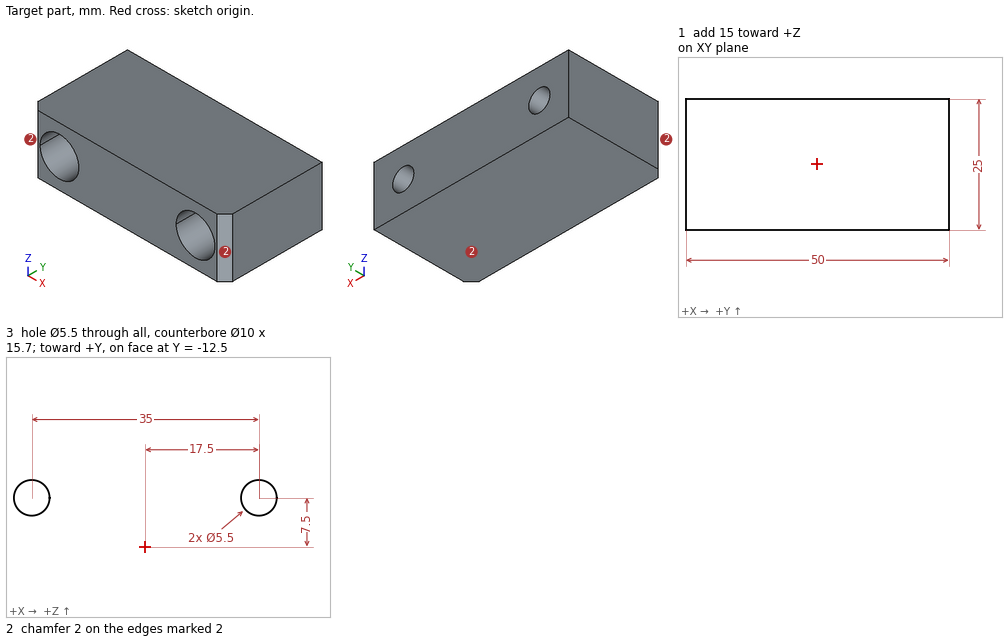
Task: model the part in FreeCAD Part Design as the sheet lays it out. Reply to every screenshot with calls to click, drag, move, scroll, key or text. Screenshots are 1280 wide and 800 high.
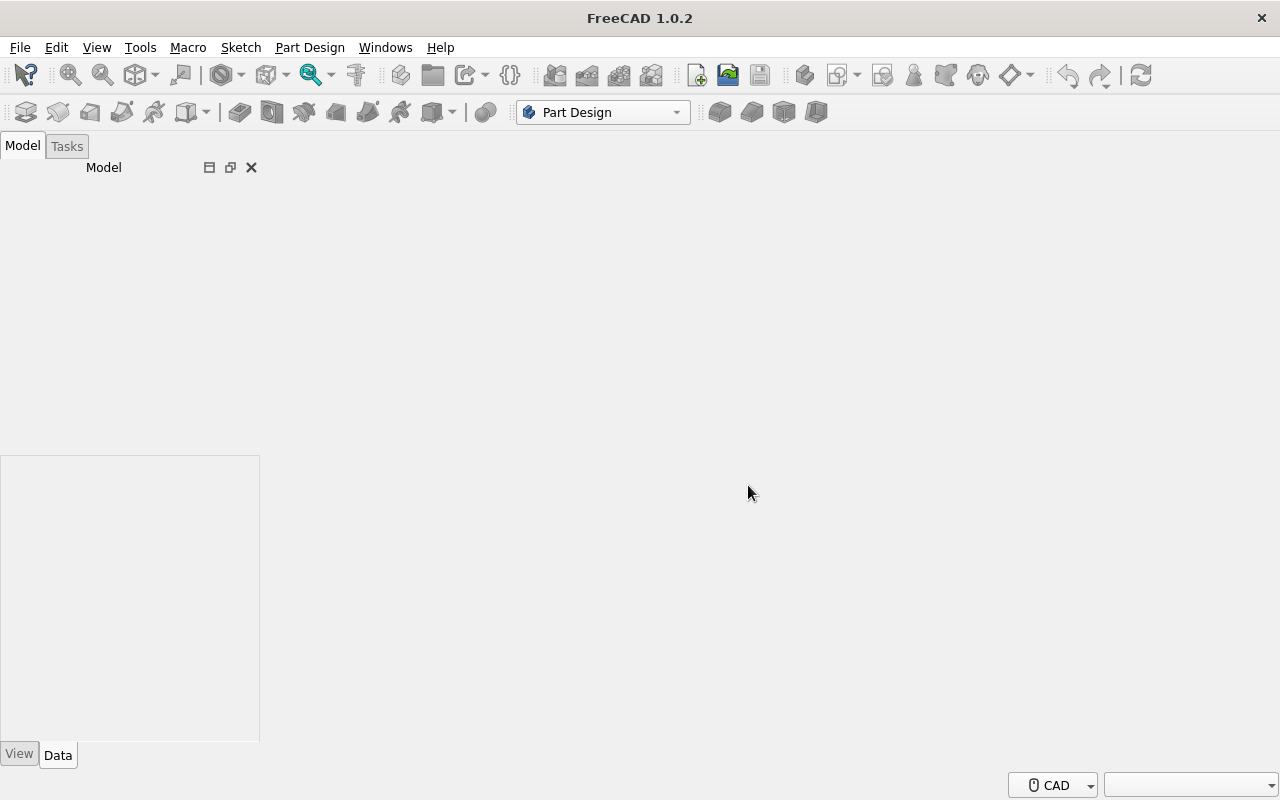
key(ctrl+n)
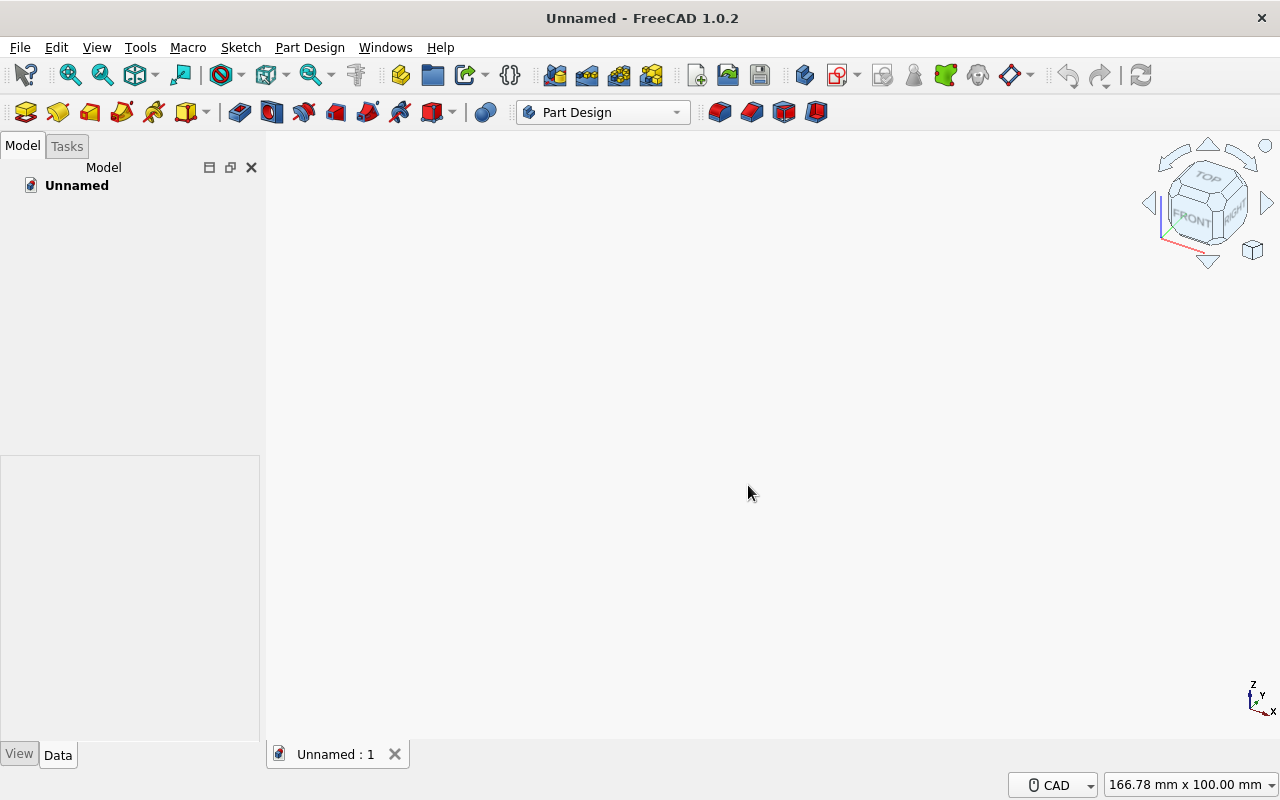
click(838, 76)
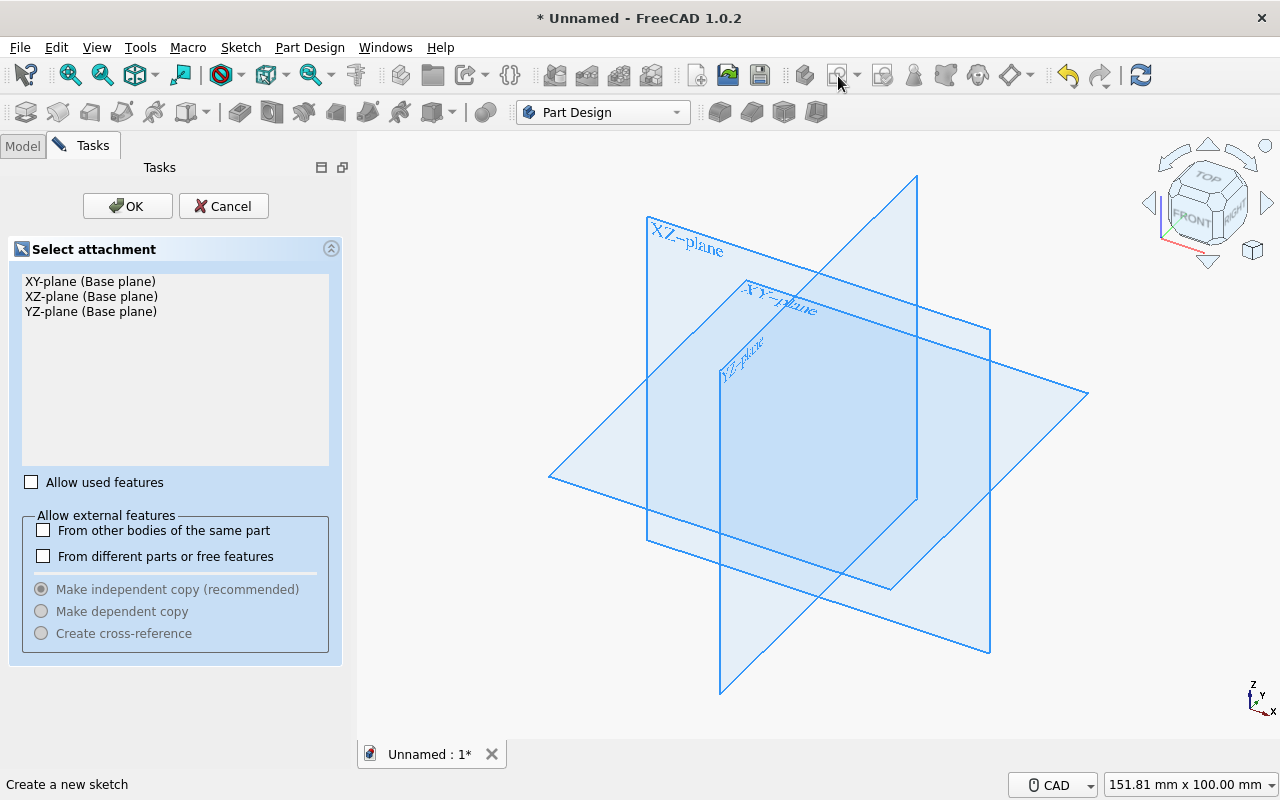
click(82, 282)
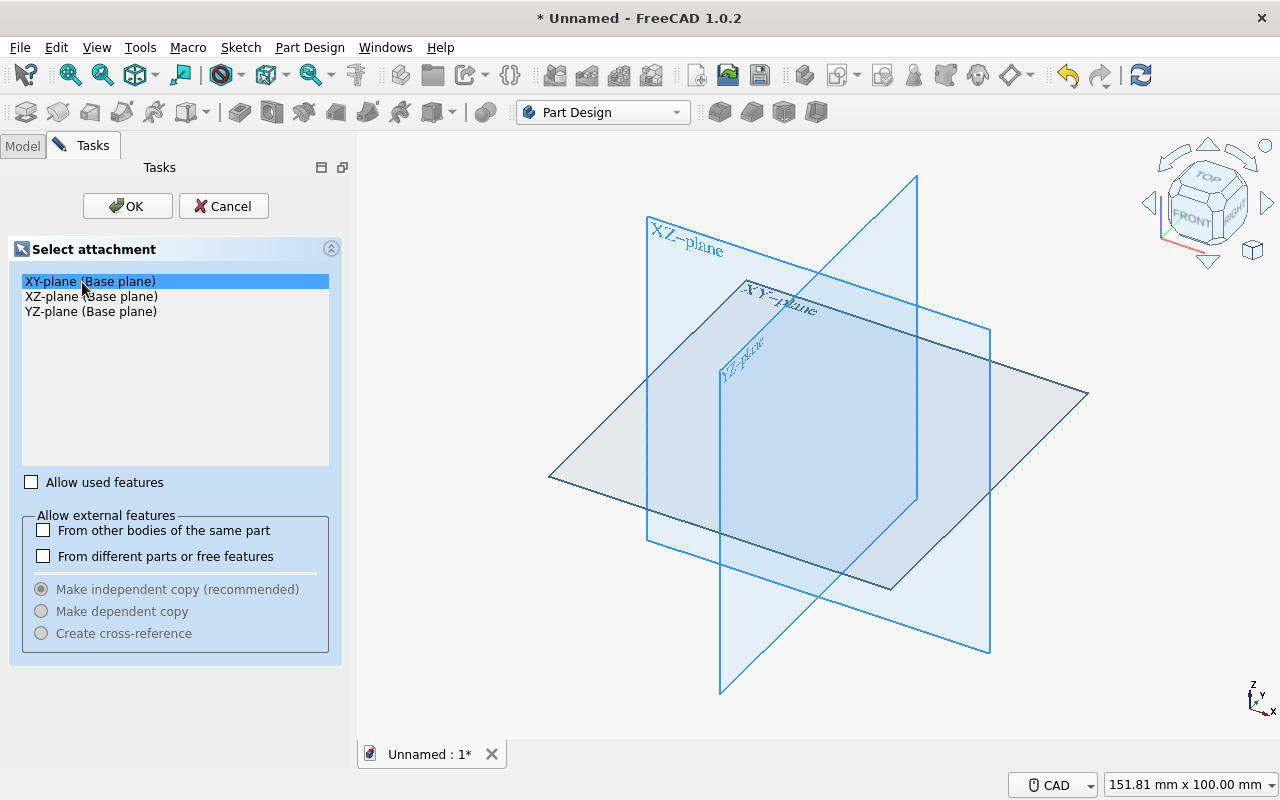
click(128, 206)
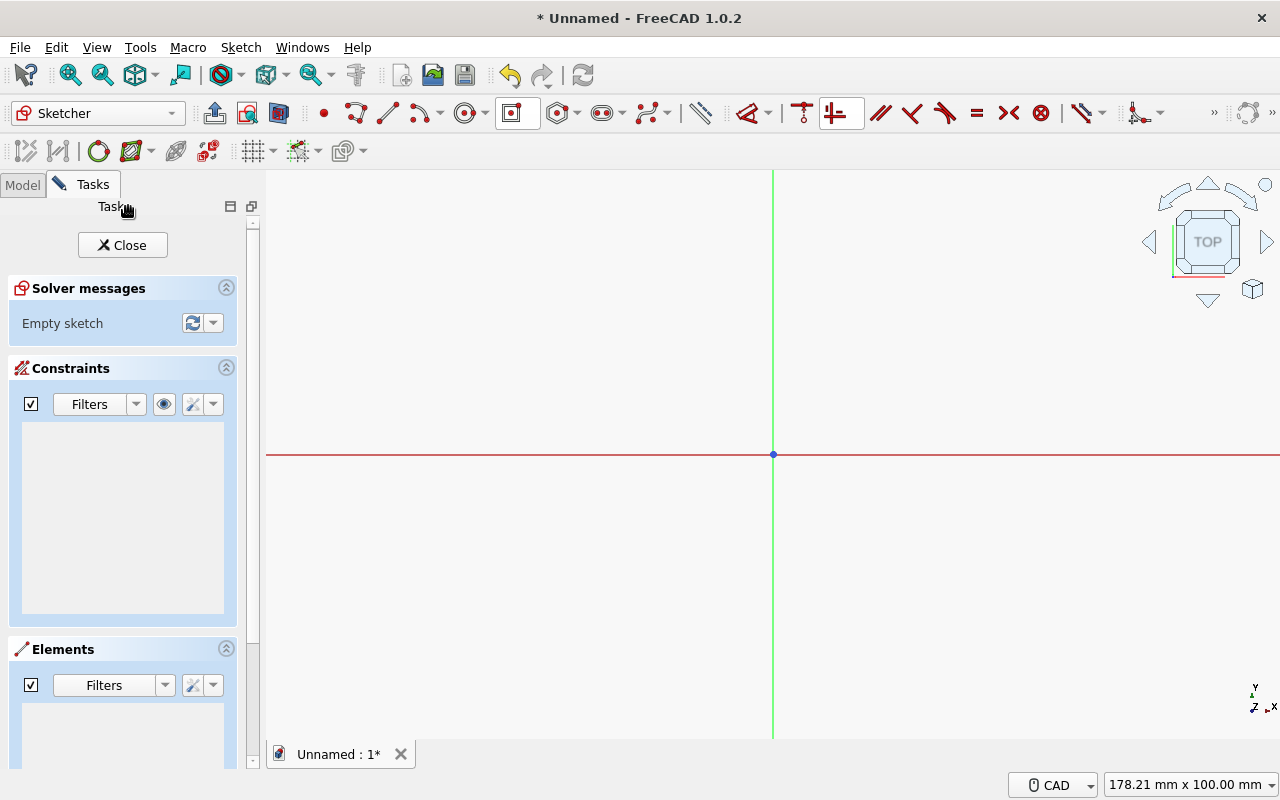
scroll(829, 455, up, 4)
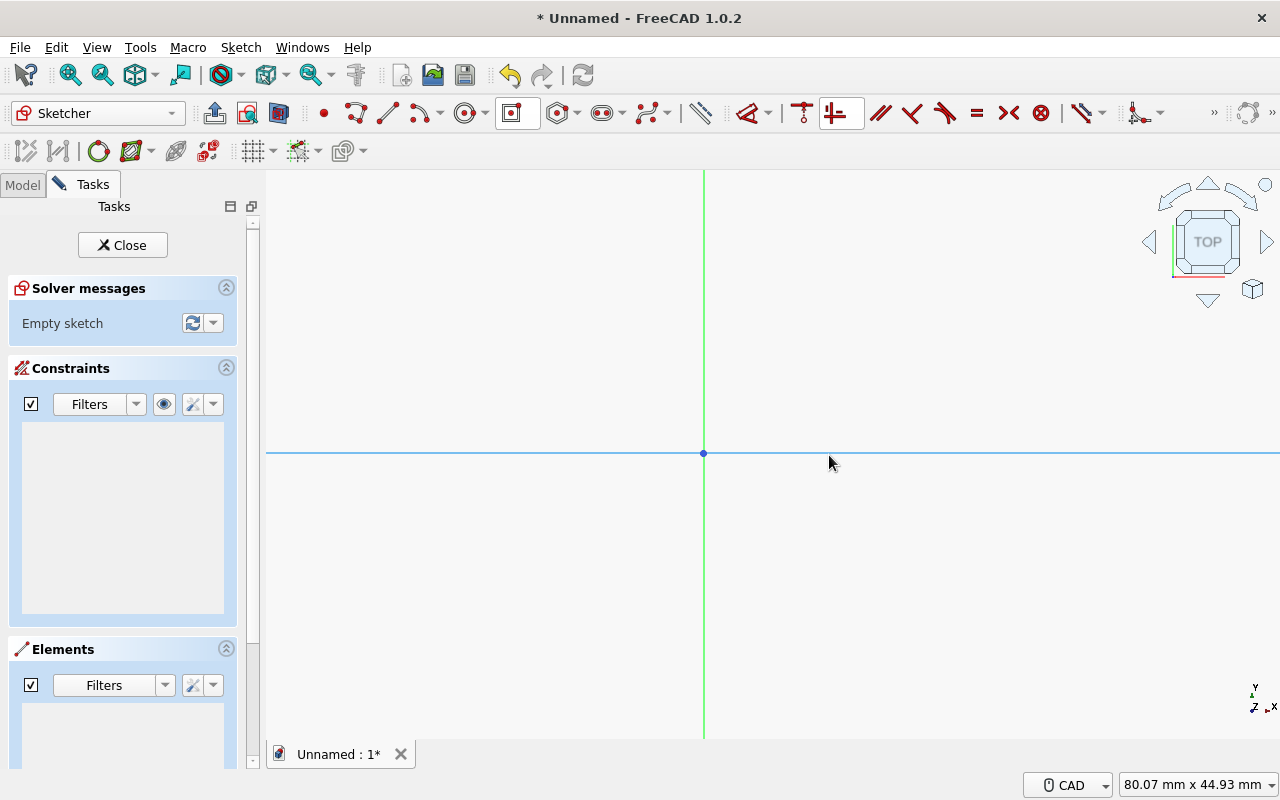
key(g)
key(v)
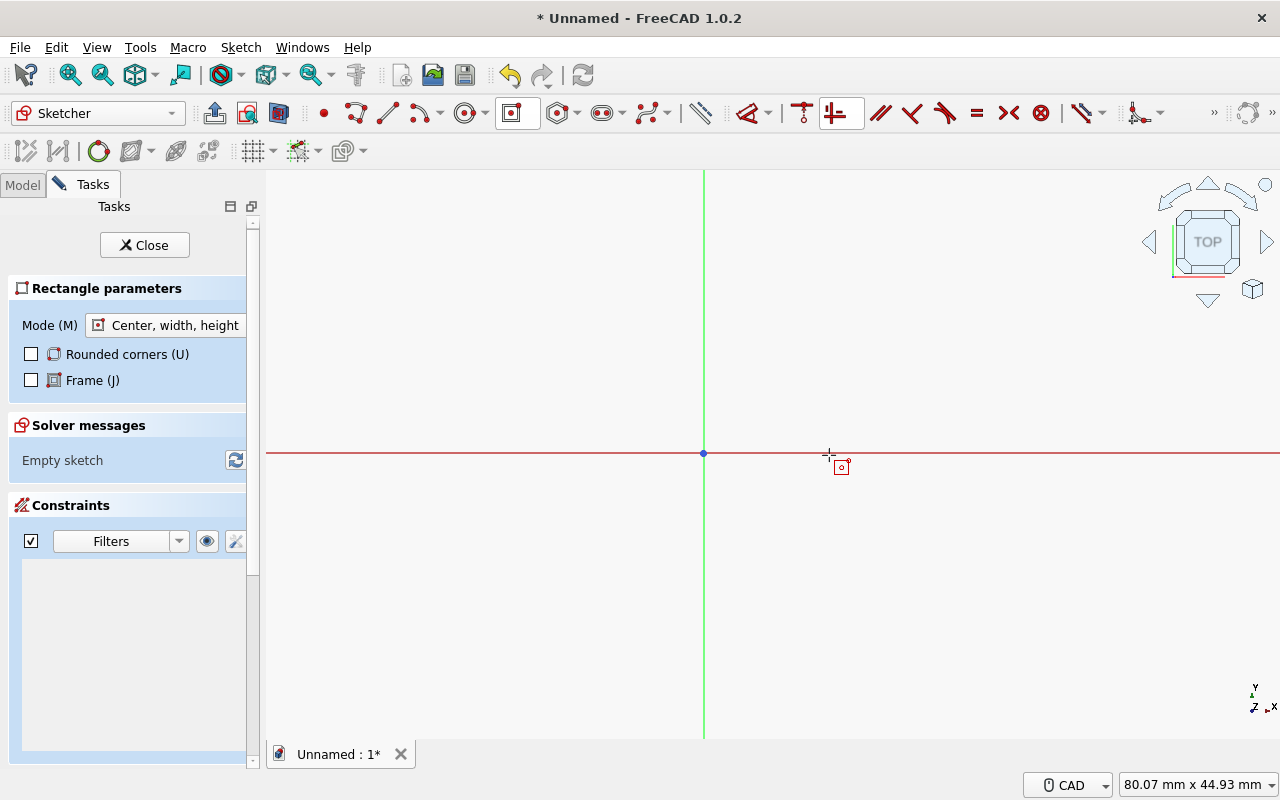
click(704, 453)
move(1020, 295)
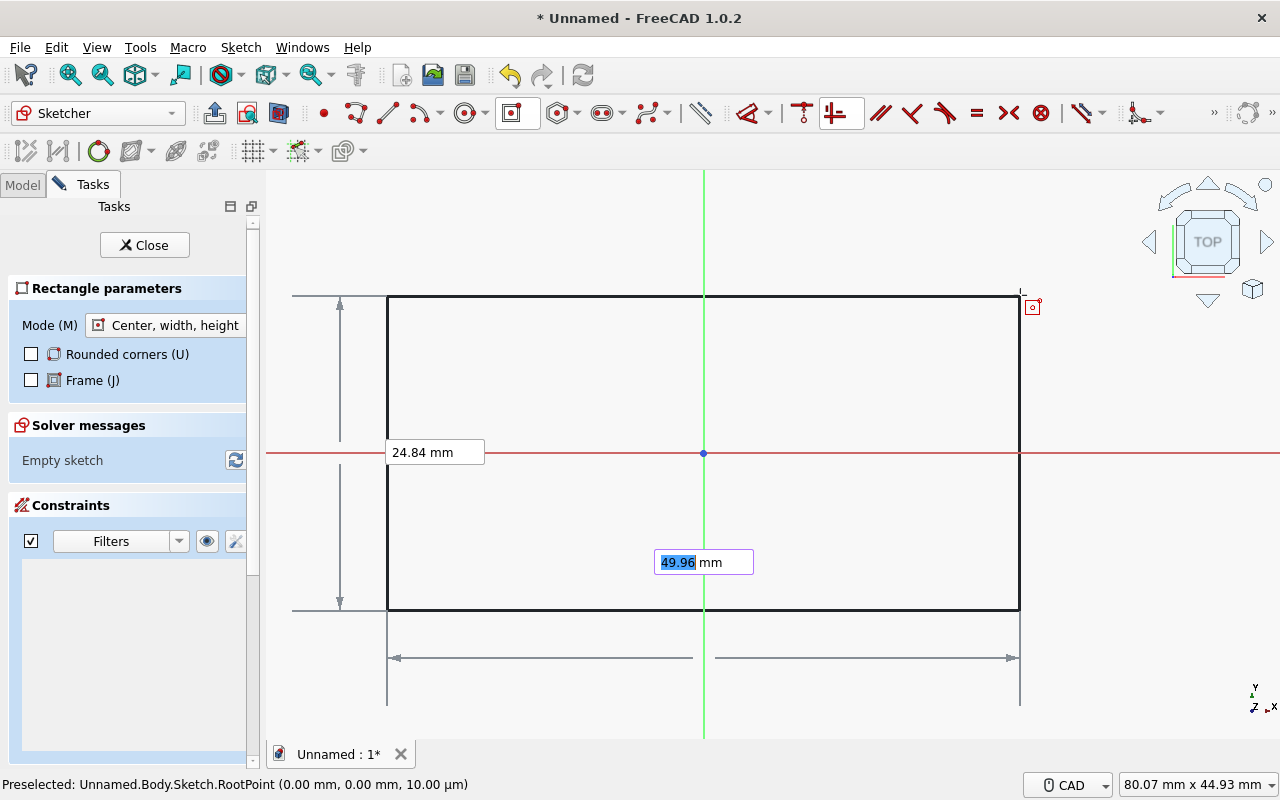
text(50)
key(Tab)
text(25)
key(Return)
key(Escape)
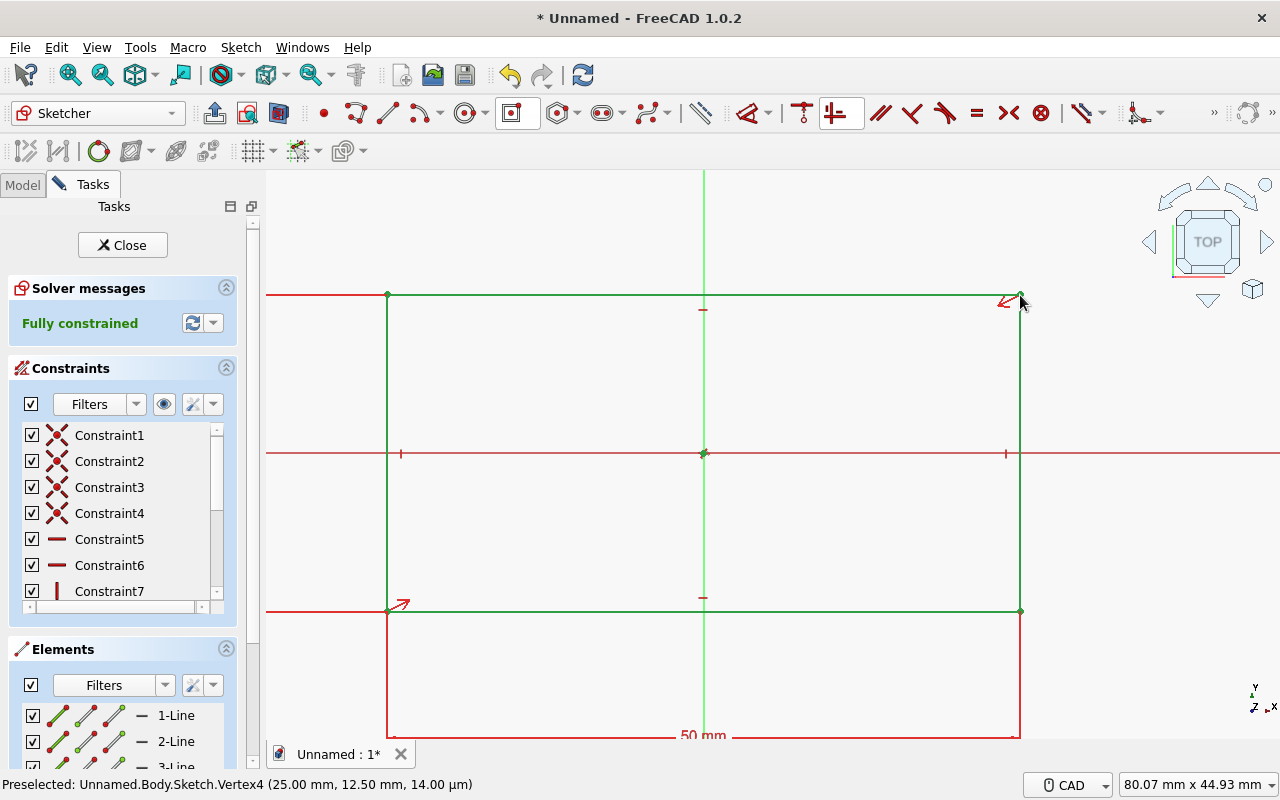
click(123, 245)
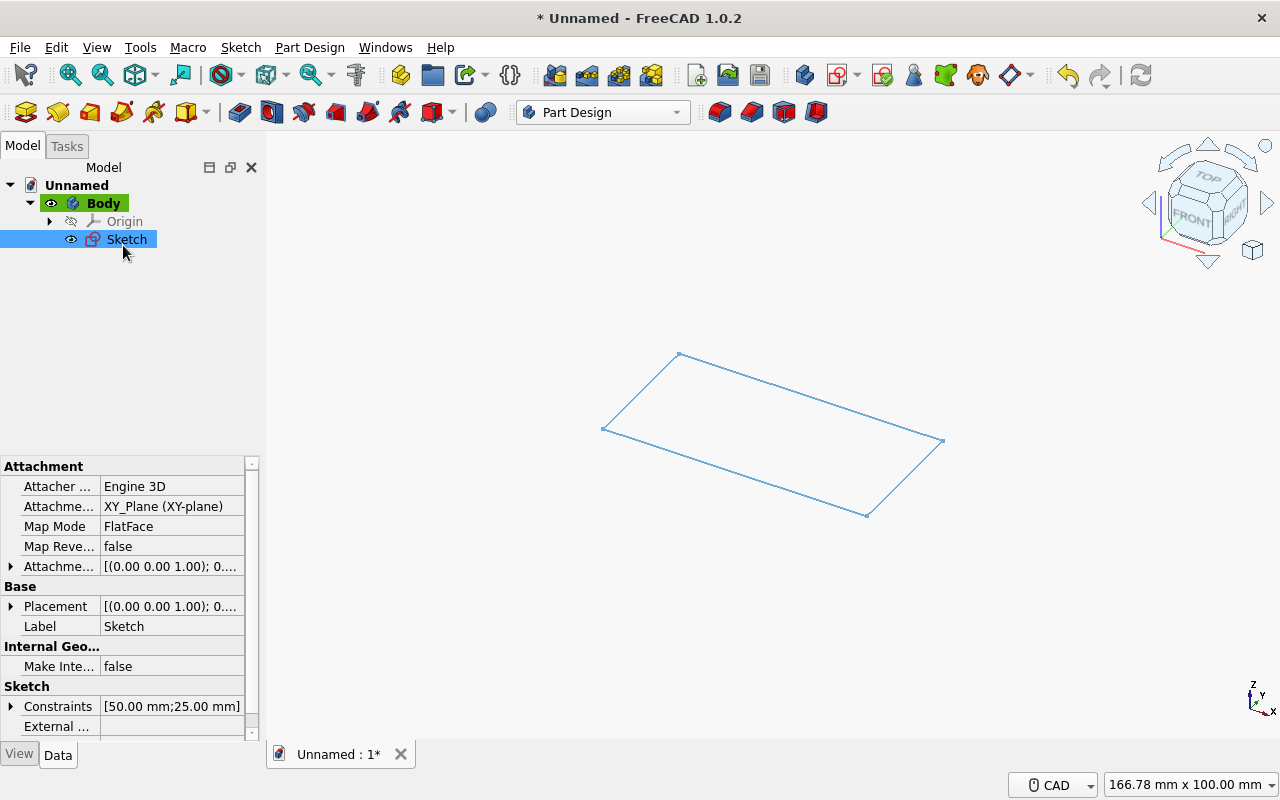
click(26, 112)